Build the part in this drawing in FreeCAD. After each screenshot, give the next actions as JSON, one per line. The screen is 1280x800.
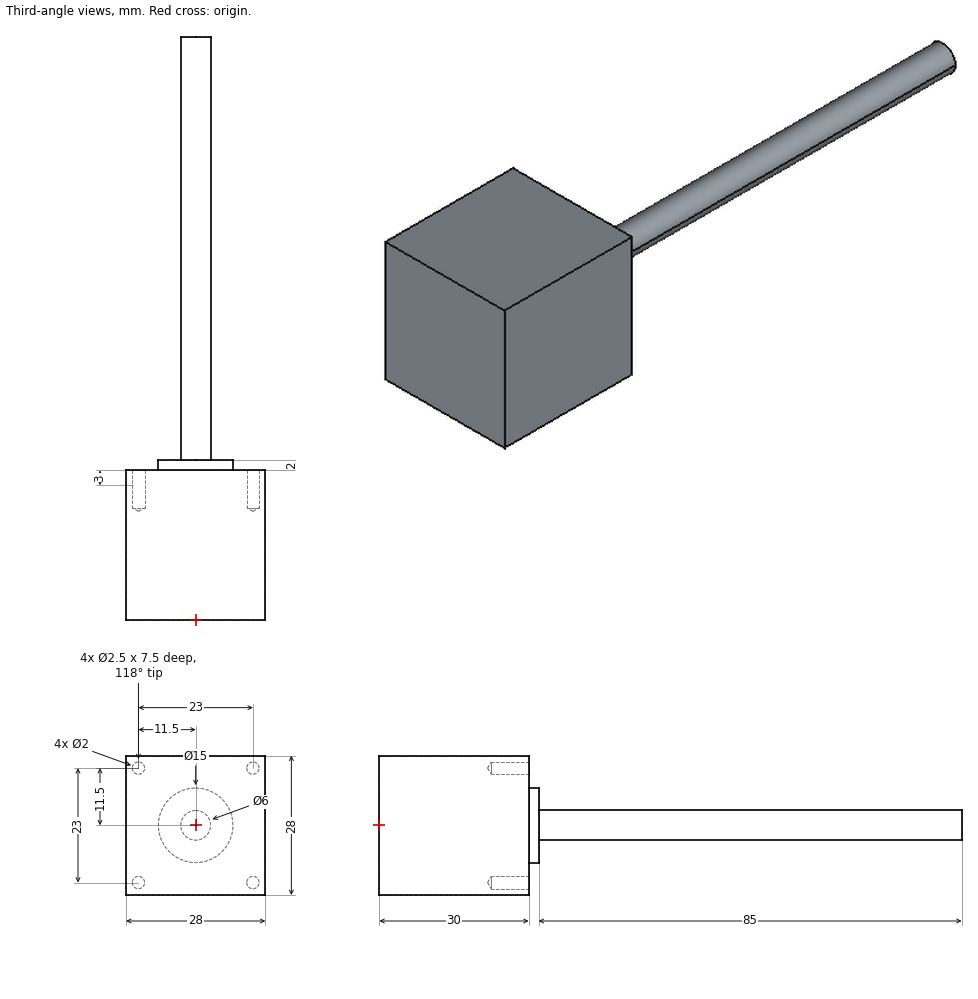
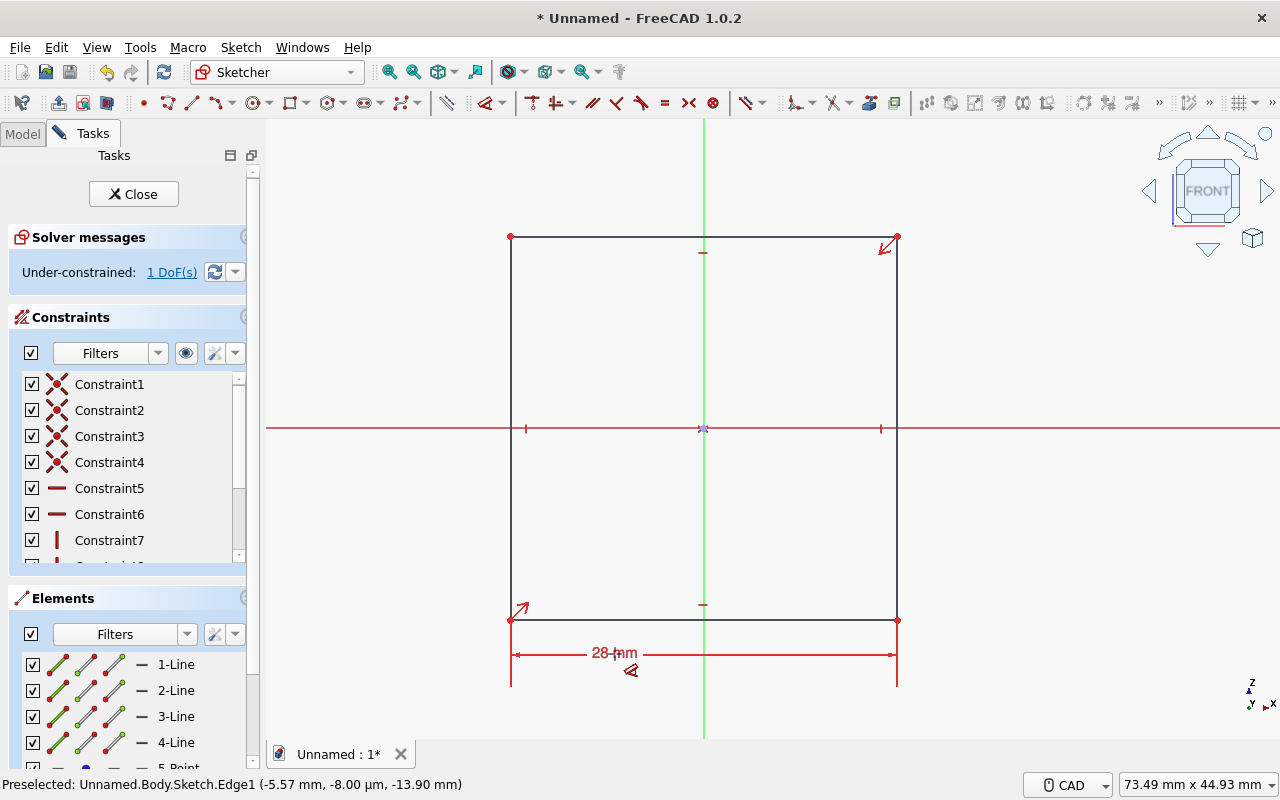
{"action": "left_click", "coordinate": [897, 505]}
{"action": "left_click", "coordinate": [931, 340]}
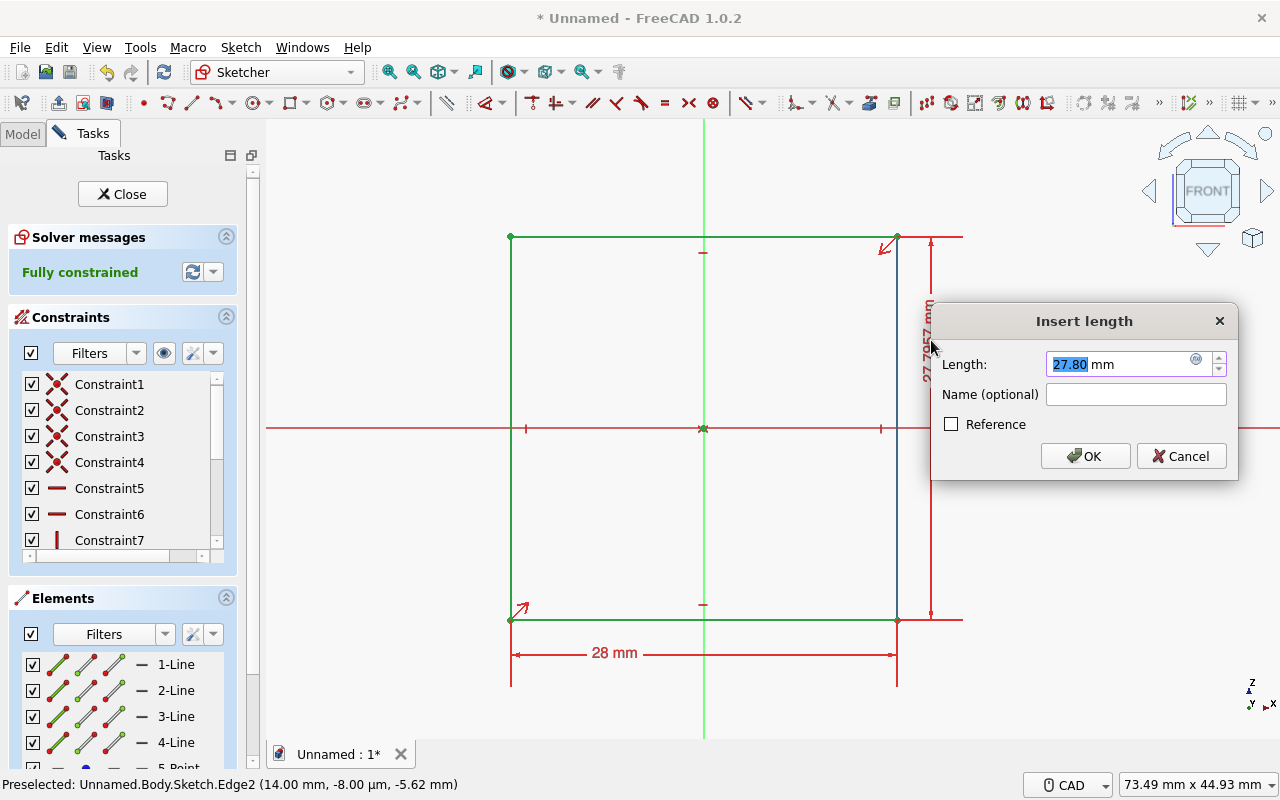
{"action": "type", "text": "28"}
{"action": "key", "text": "Return"}
{"action": "key", "text": "Escape"}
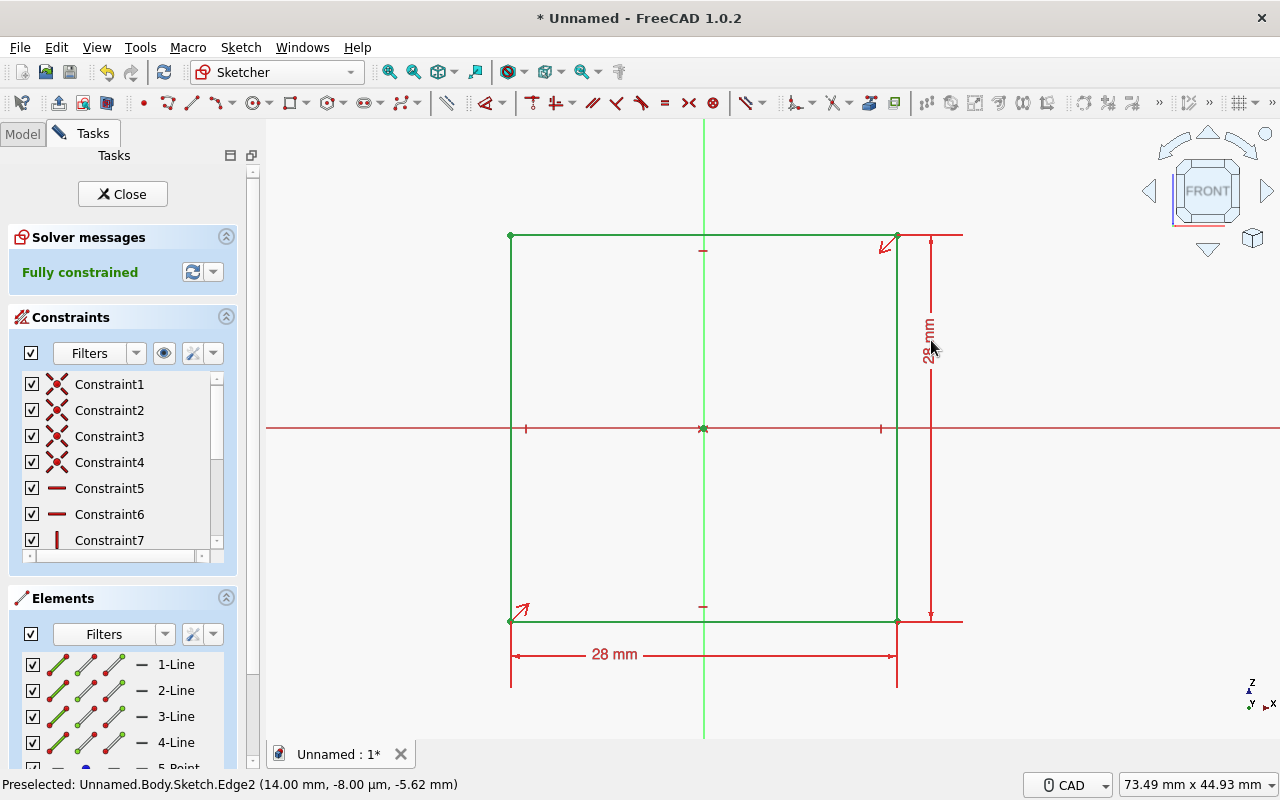
{"action": "left_click", "coordinate": [123, 194]}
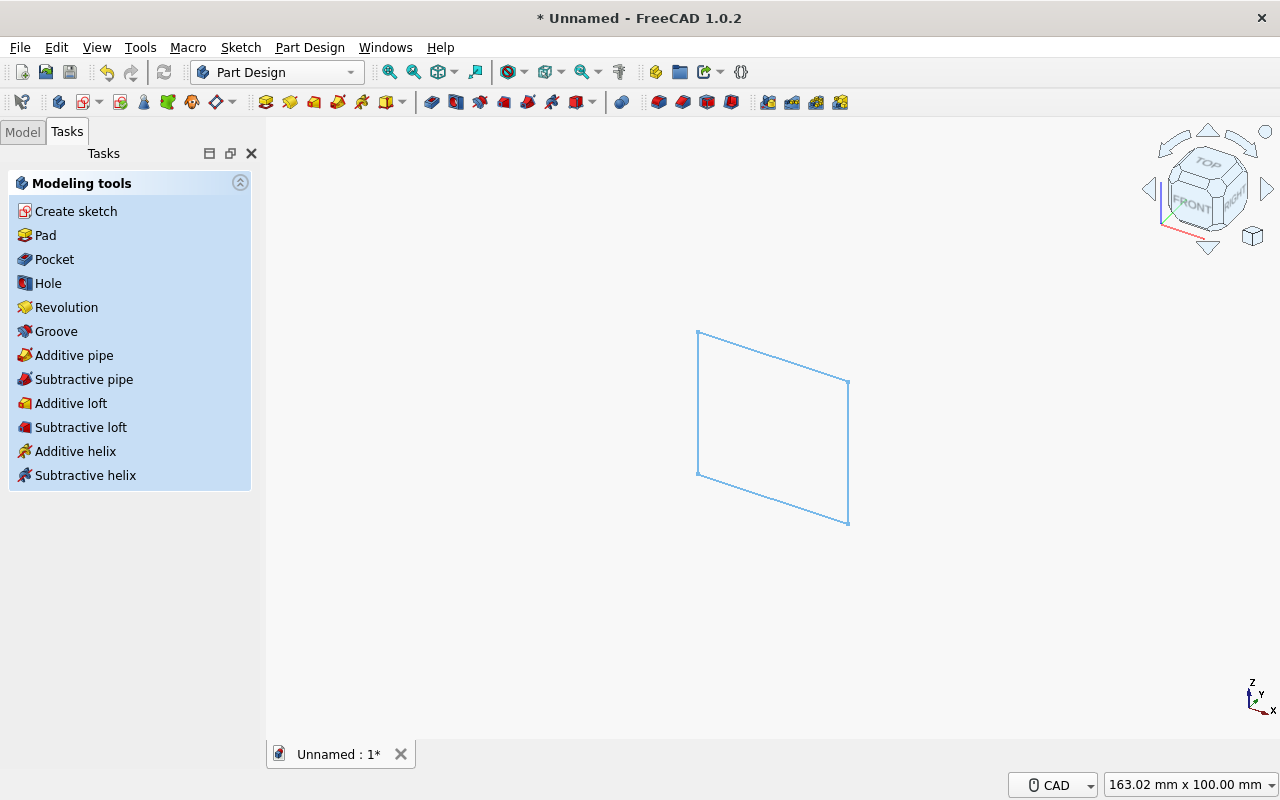
{"action": "left_click", "coordinate": [266, 102]}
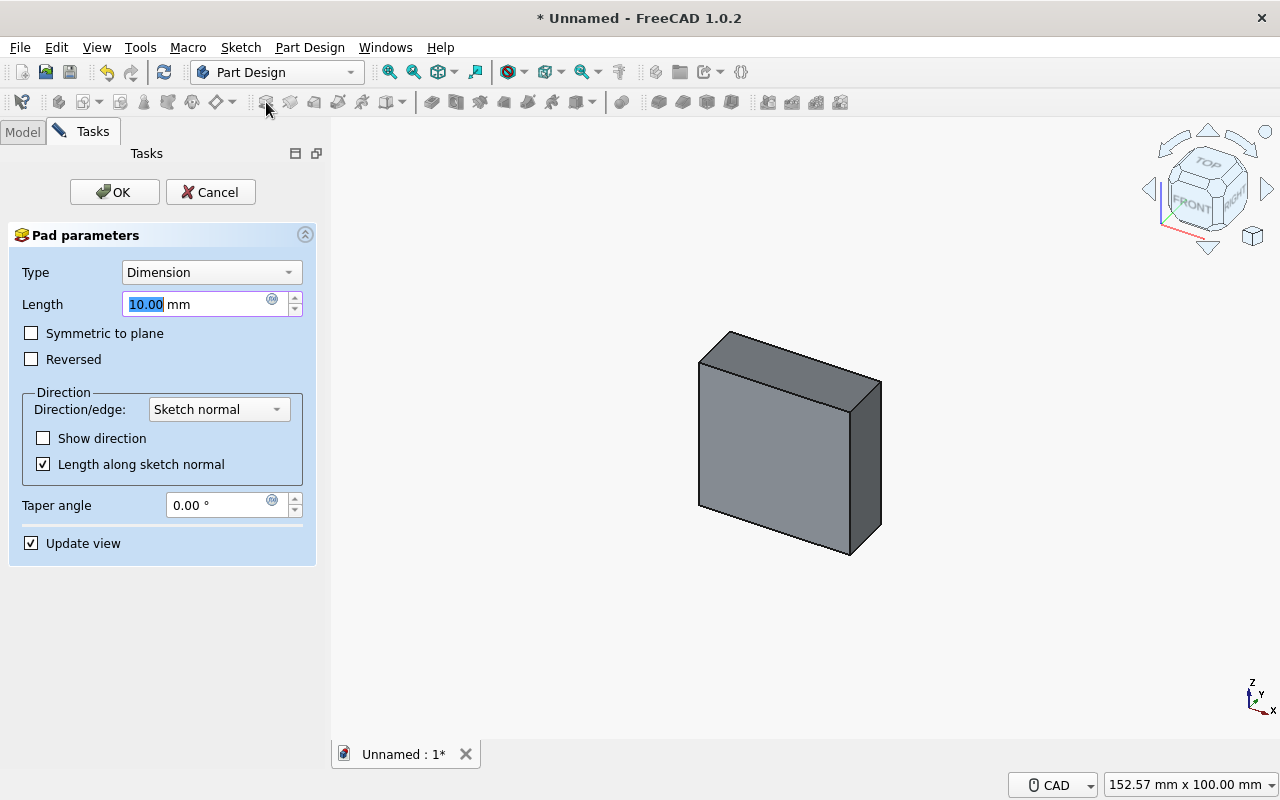
{"action": "type", "text": "30"}
{"action": "key", "text": "Tab"}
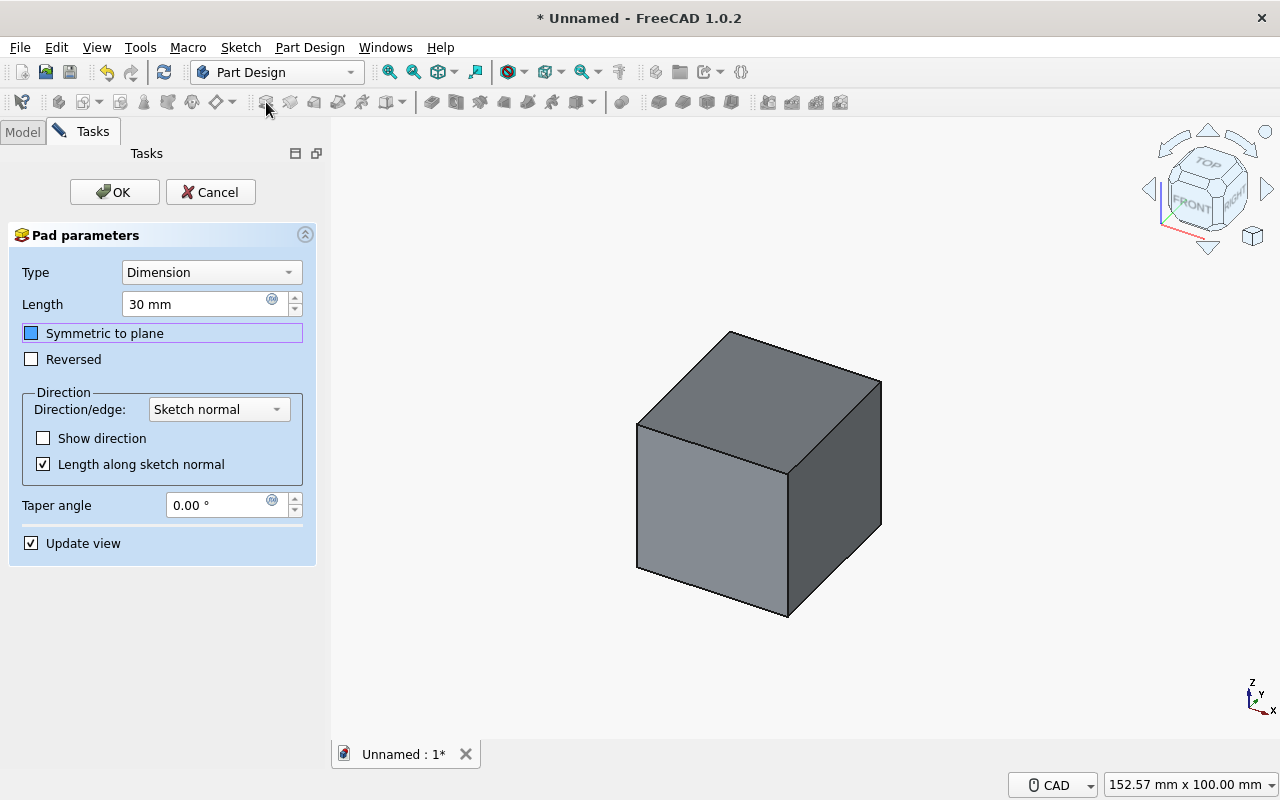
{"action": "left_click", "coordinate": [30, 359]}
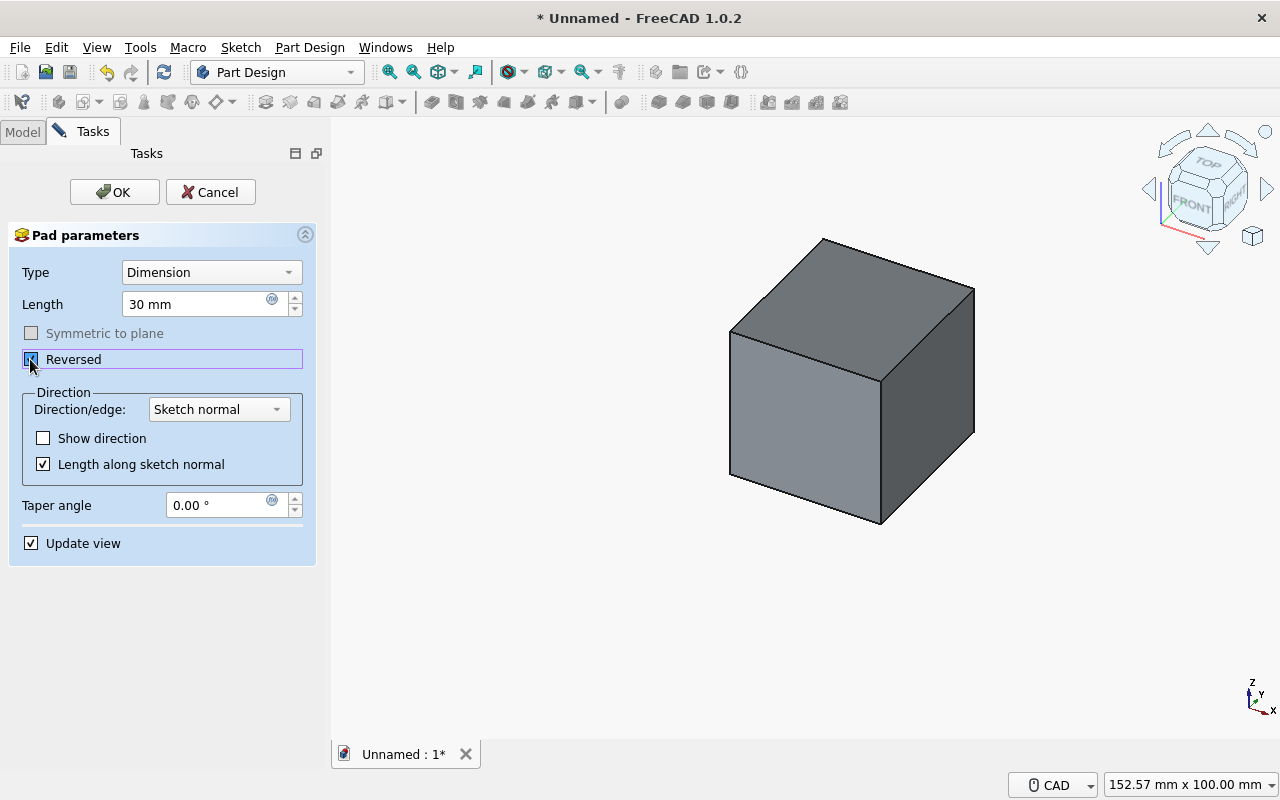
{"action": "left_click", "coordinate": [115, 192]}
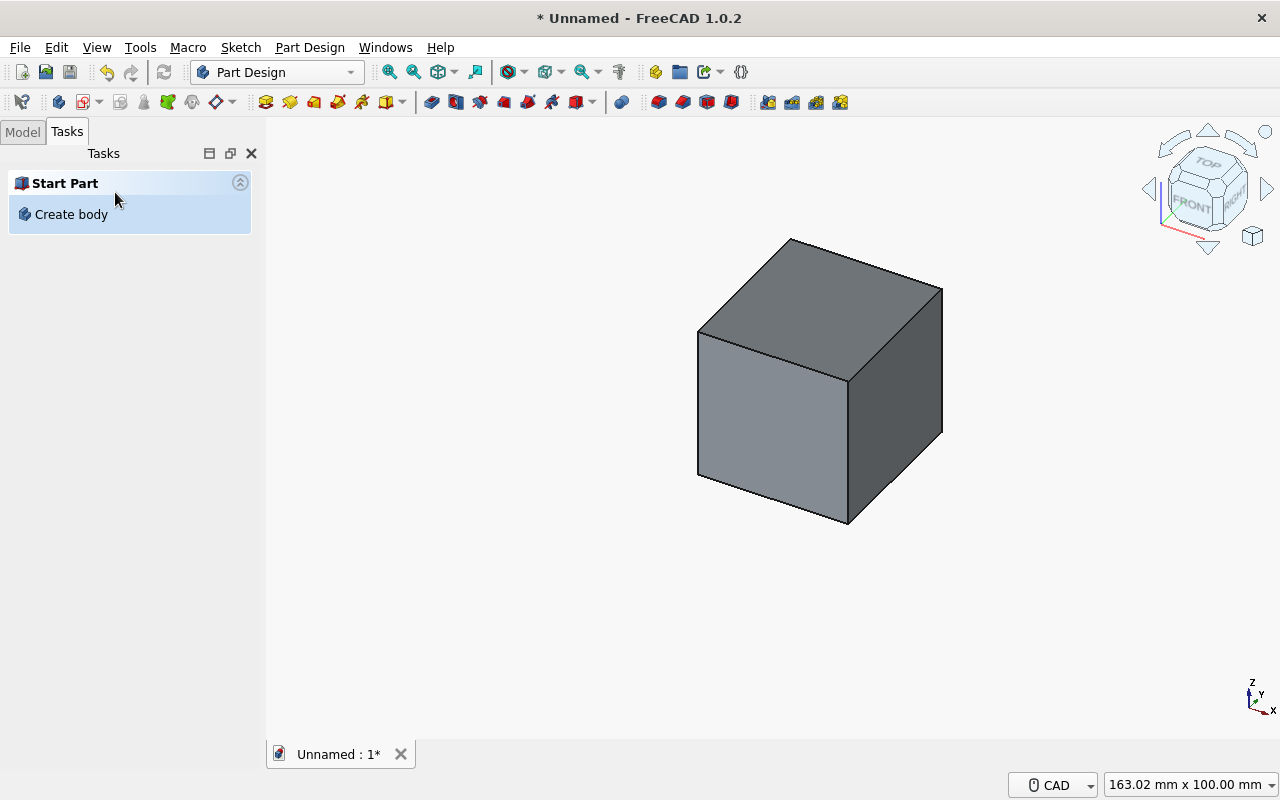
{"action": "key", "text": "4"}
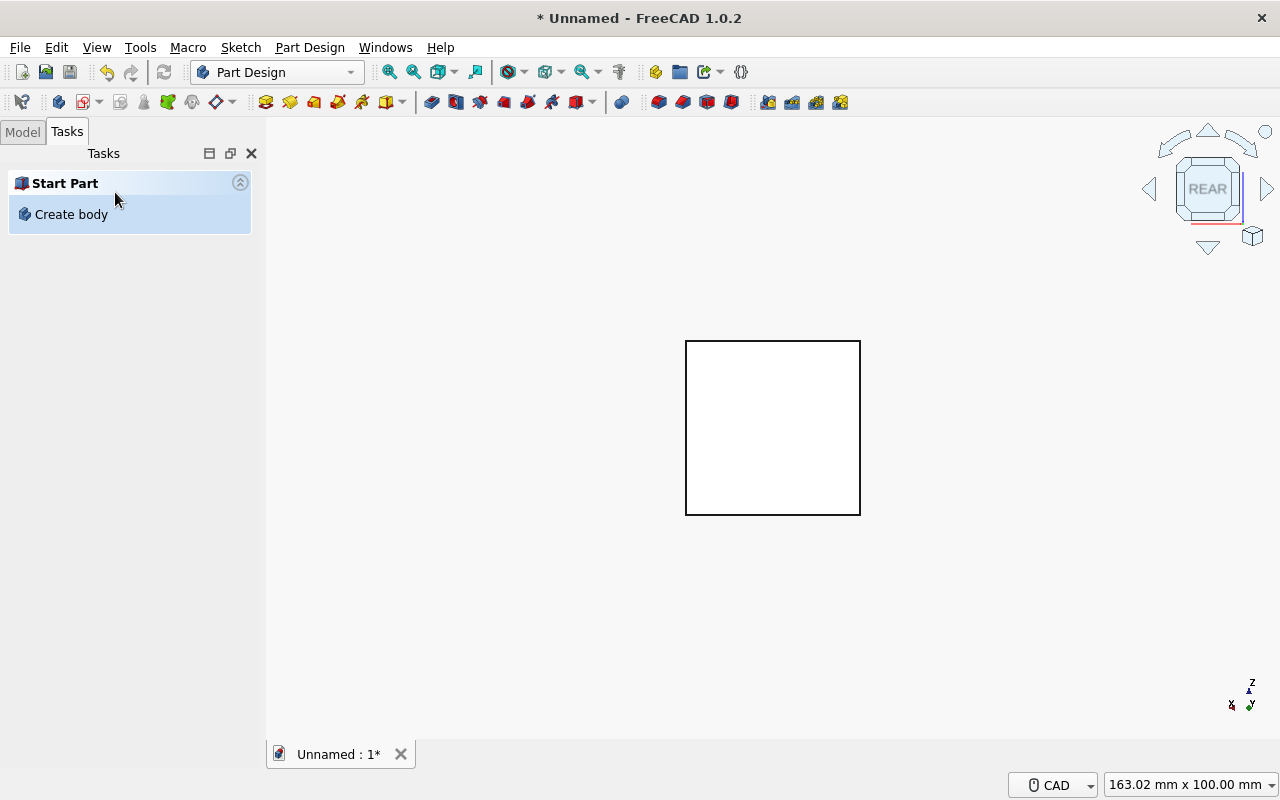
{"action": "left_click", "coordinate": [390, 72]}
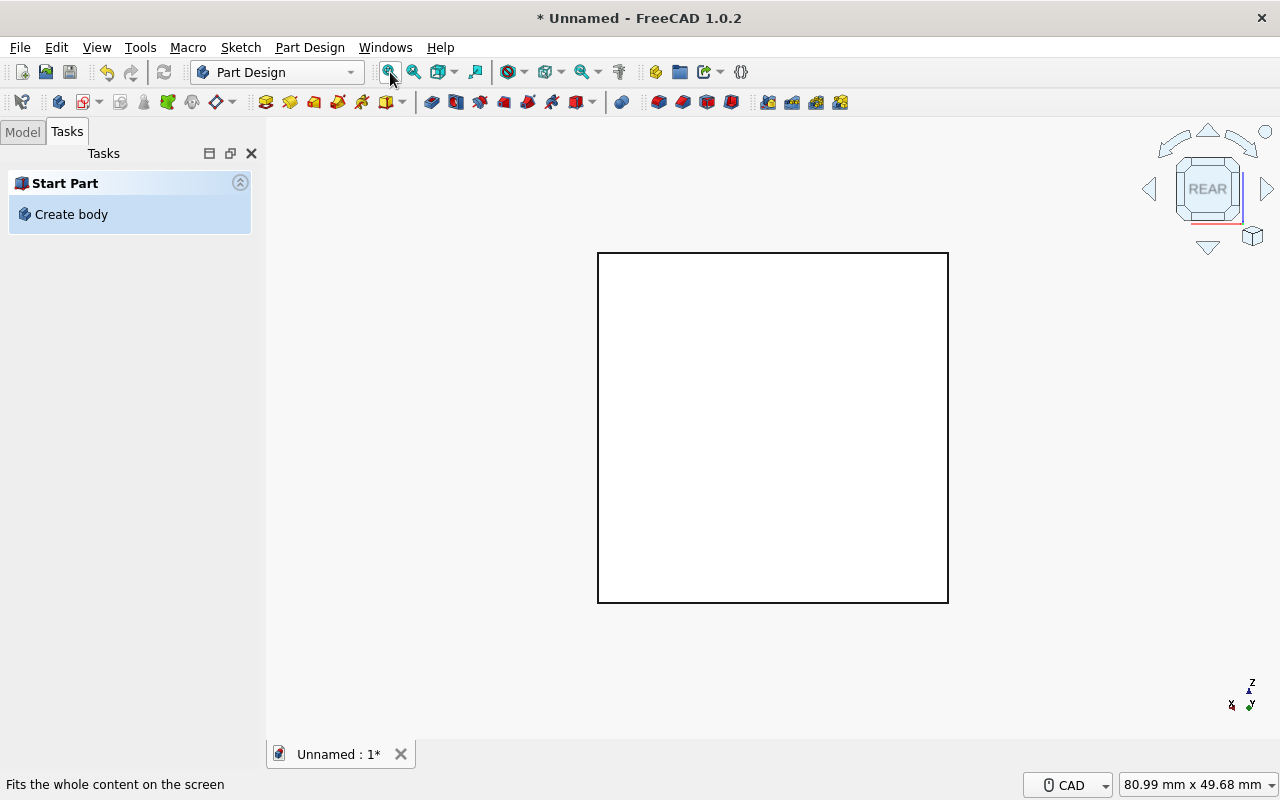
{"action": "left_click", "coordinate": [773, 427]}